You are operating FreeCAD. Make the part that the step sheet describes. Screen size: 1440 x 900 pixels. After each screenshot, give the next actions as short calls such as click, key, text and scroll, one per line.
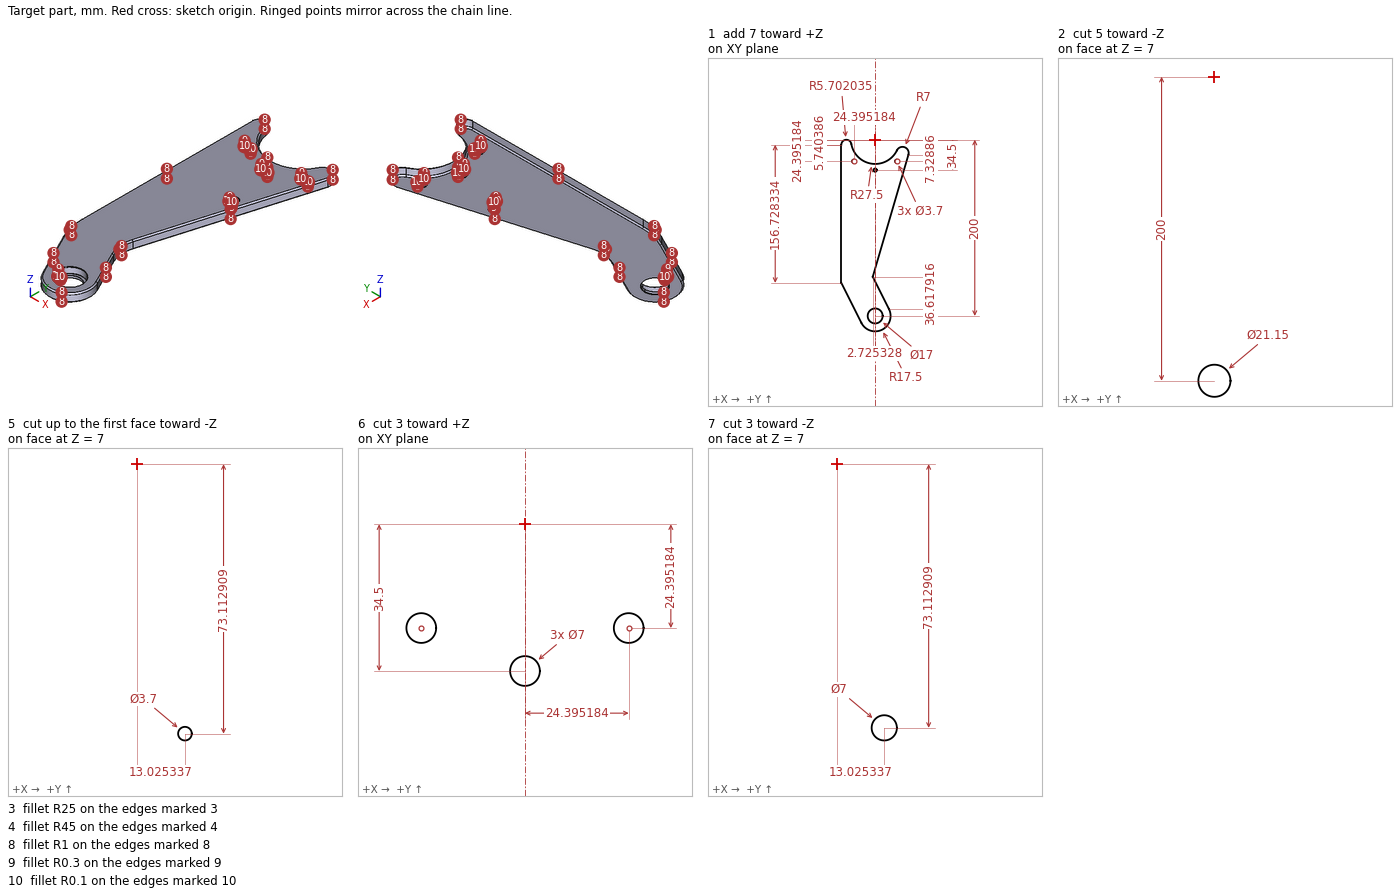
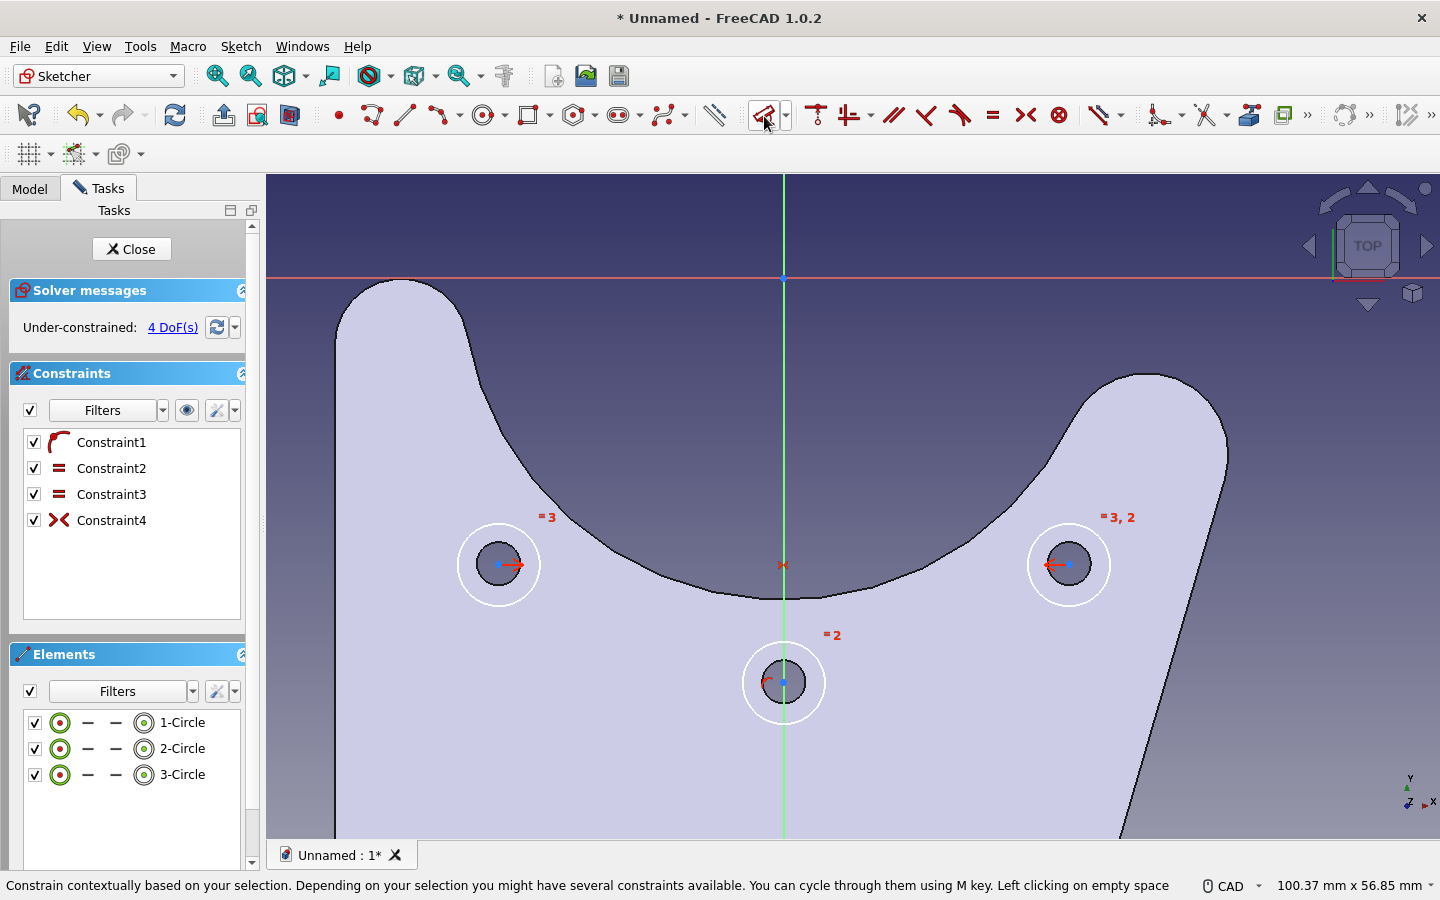
click(813, 654)
click(836, 631)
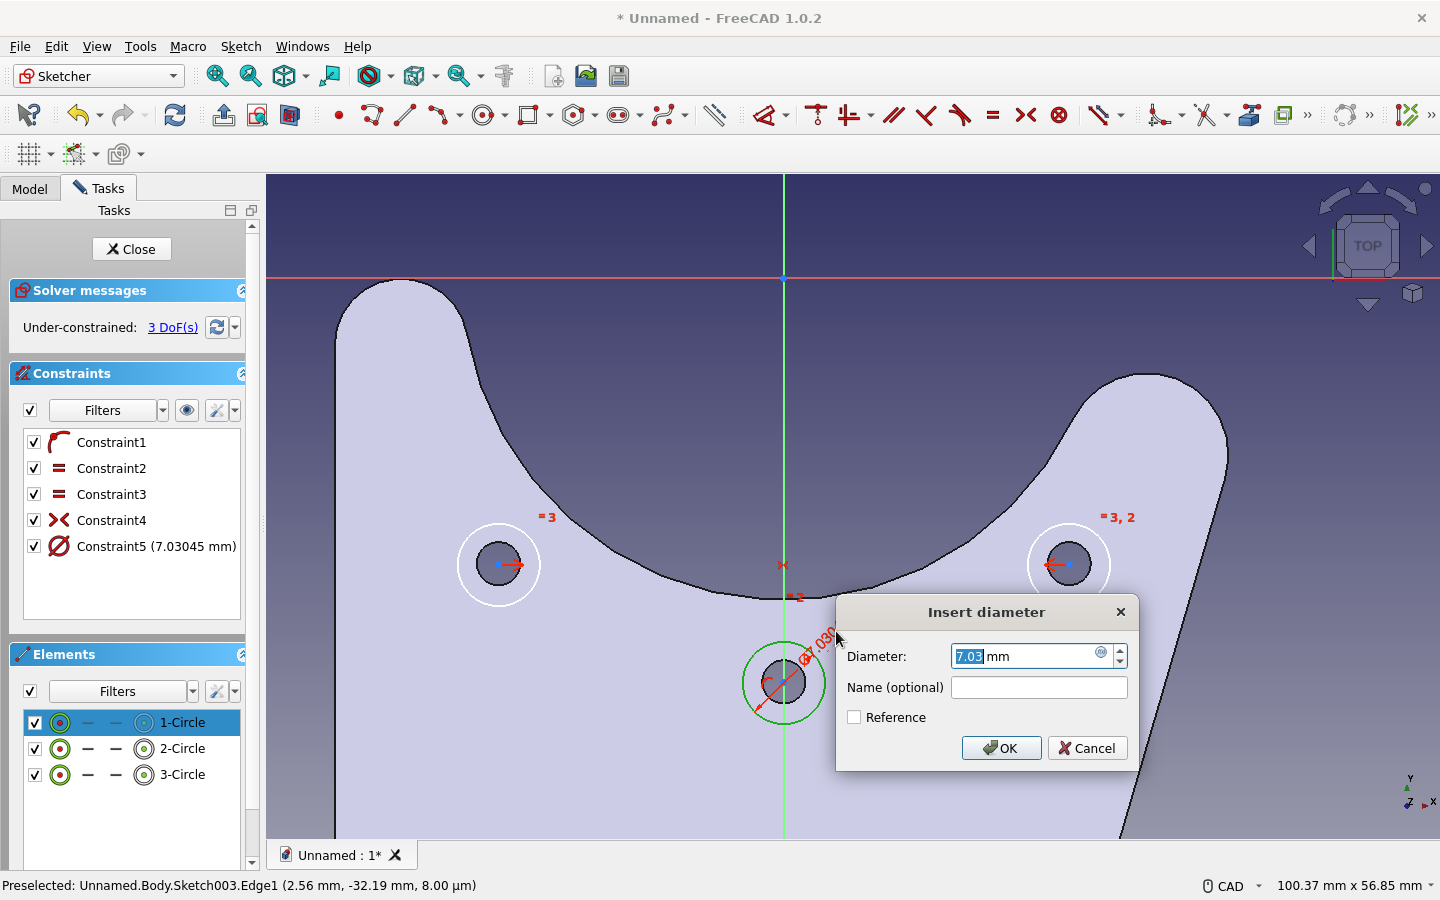
text(7)
key(Return)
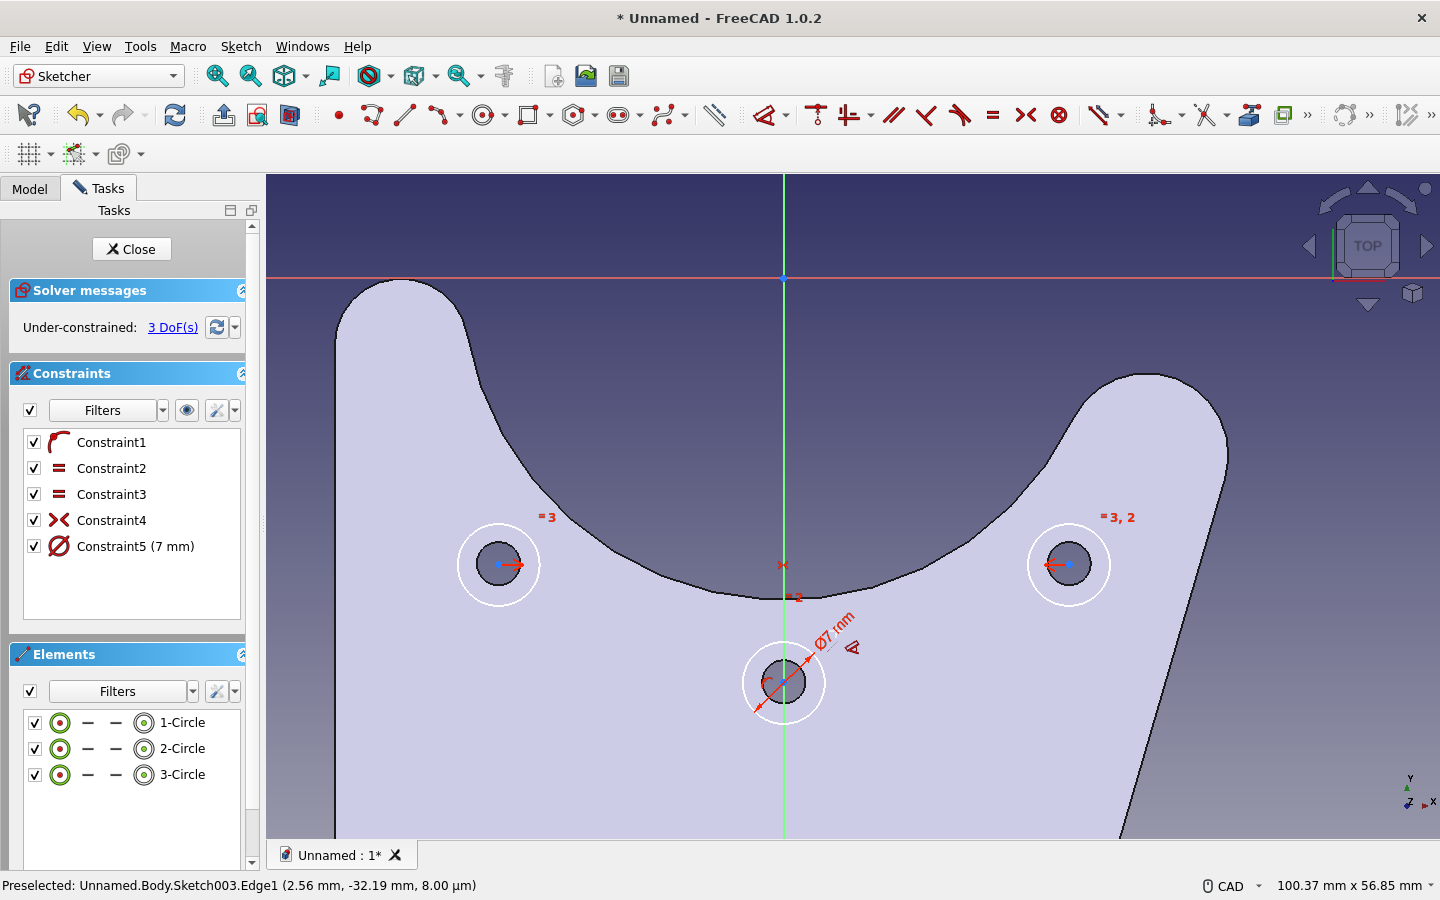
click(784, 683)
click(818, 481)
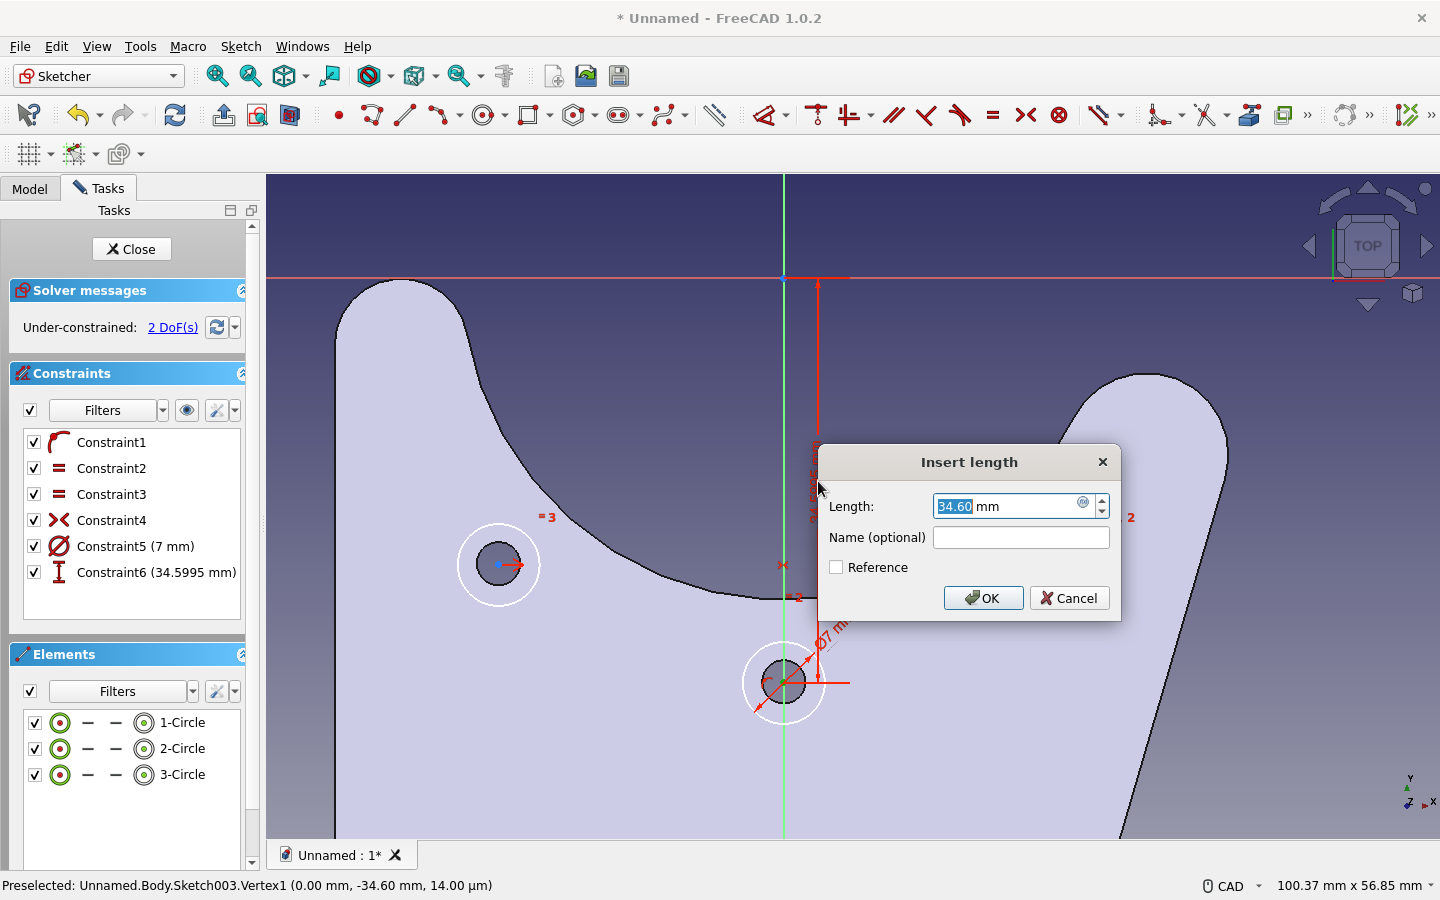
text(34.5)
key(Return)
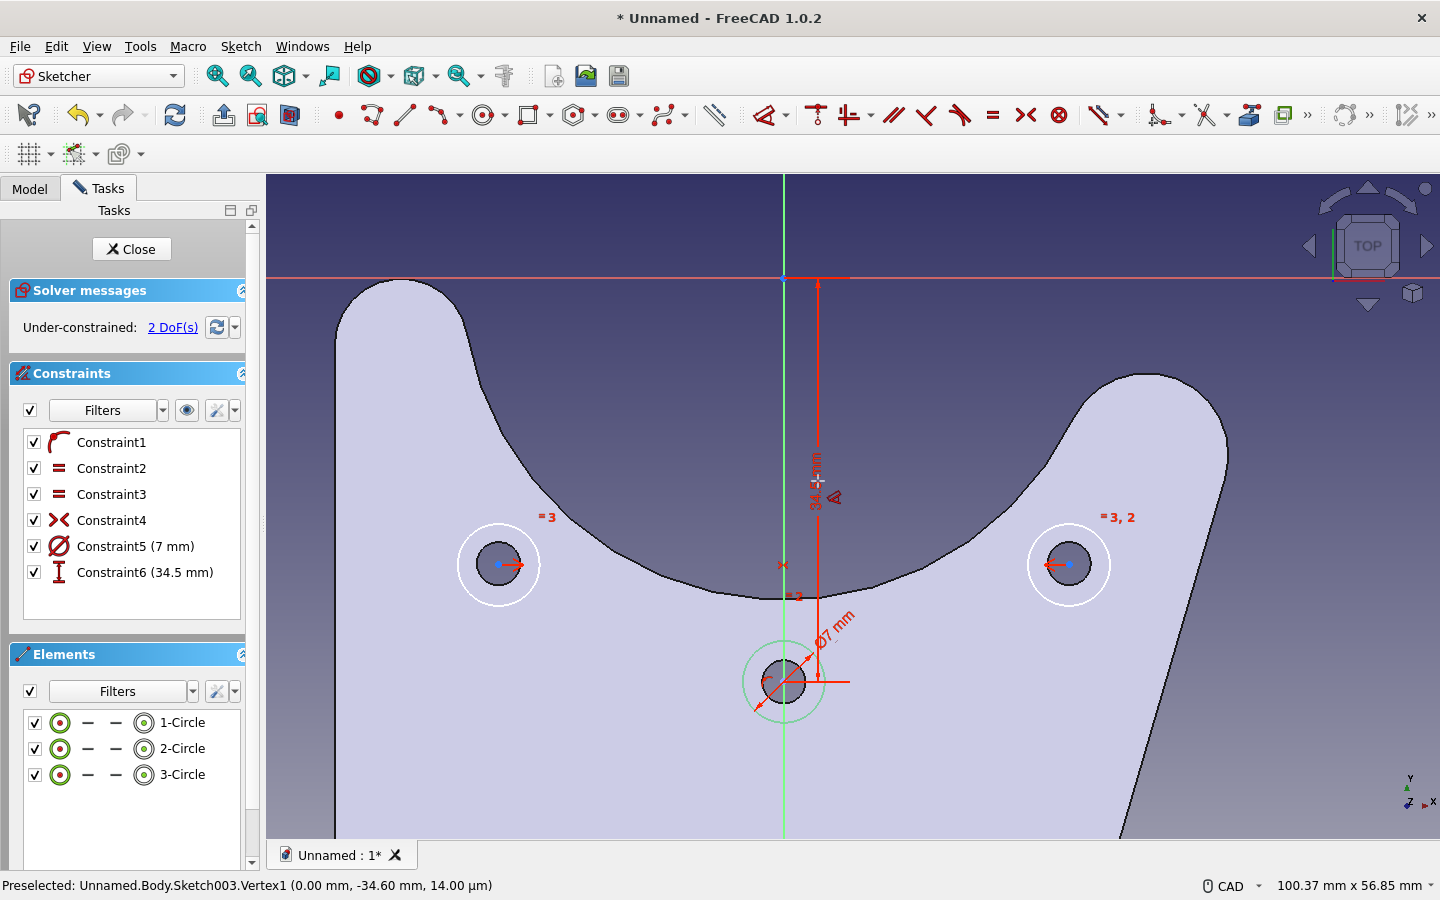
click(1069, 565)
click(926, 244)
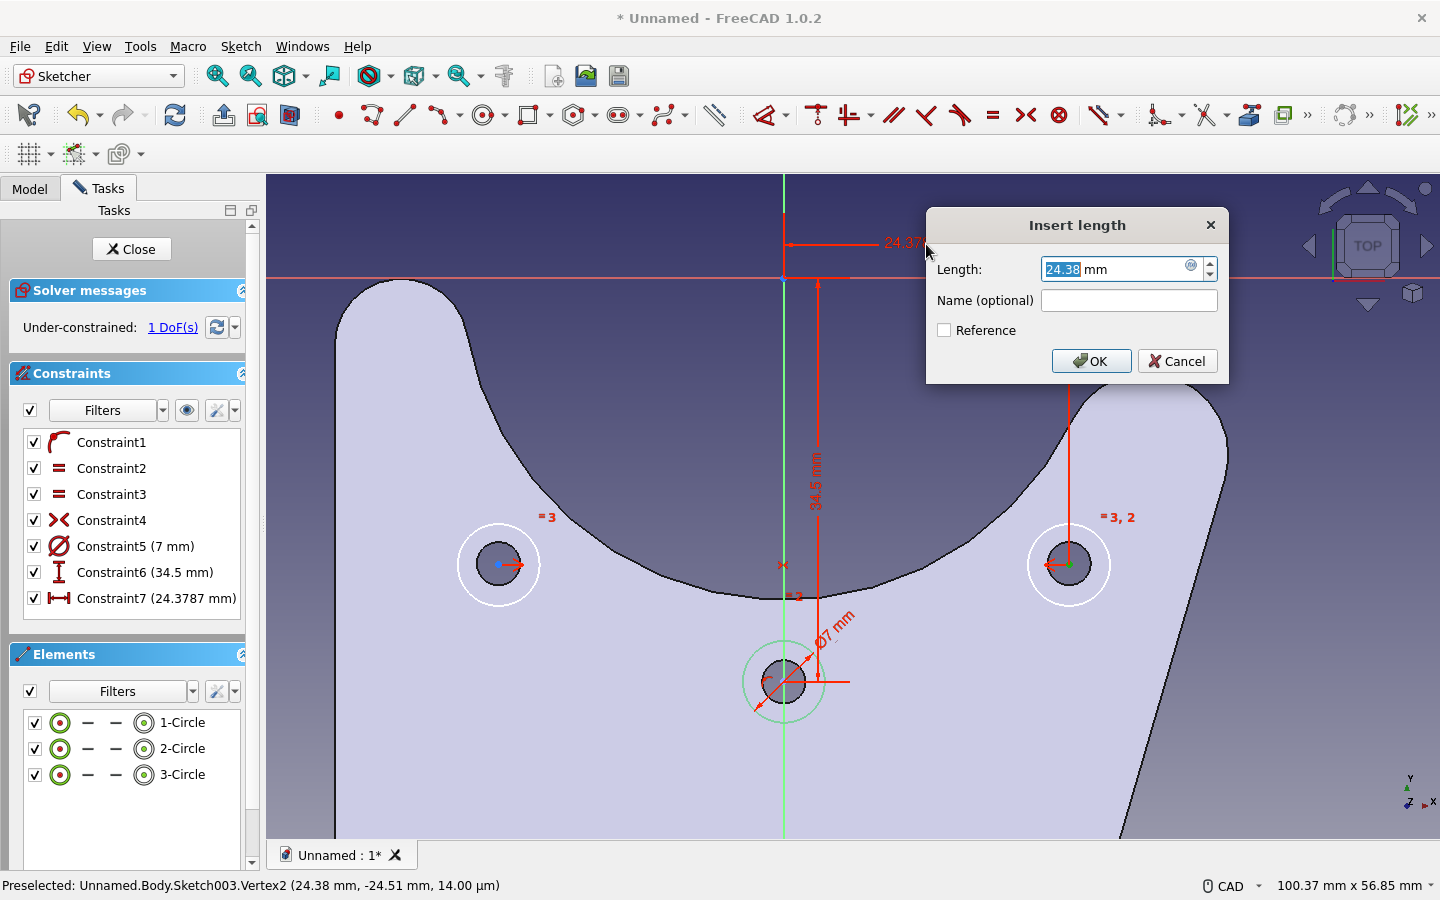
text(24.395184)
key(Return)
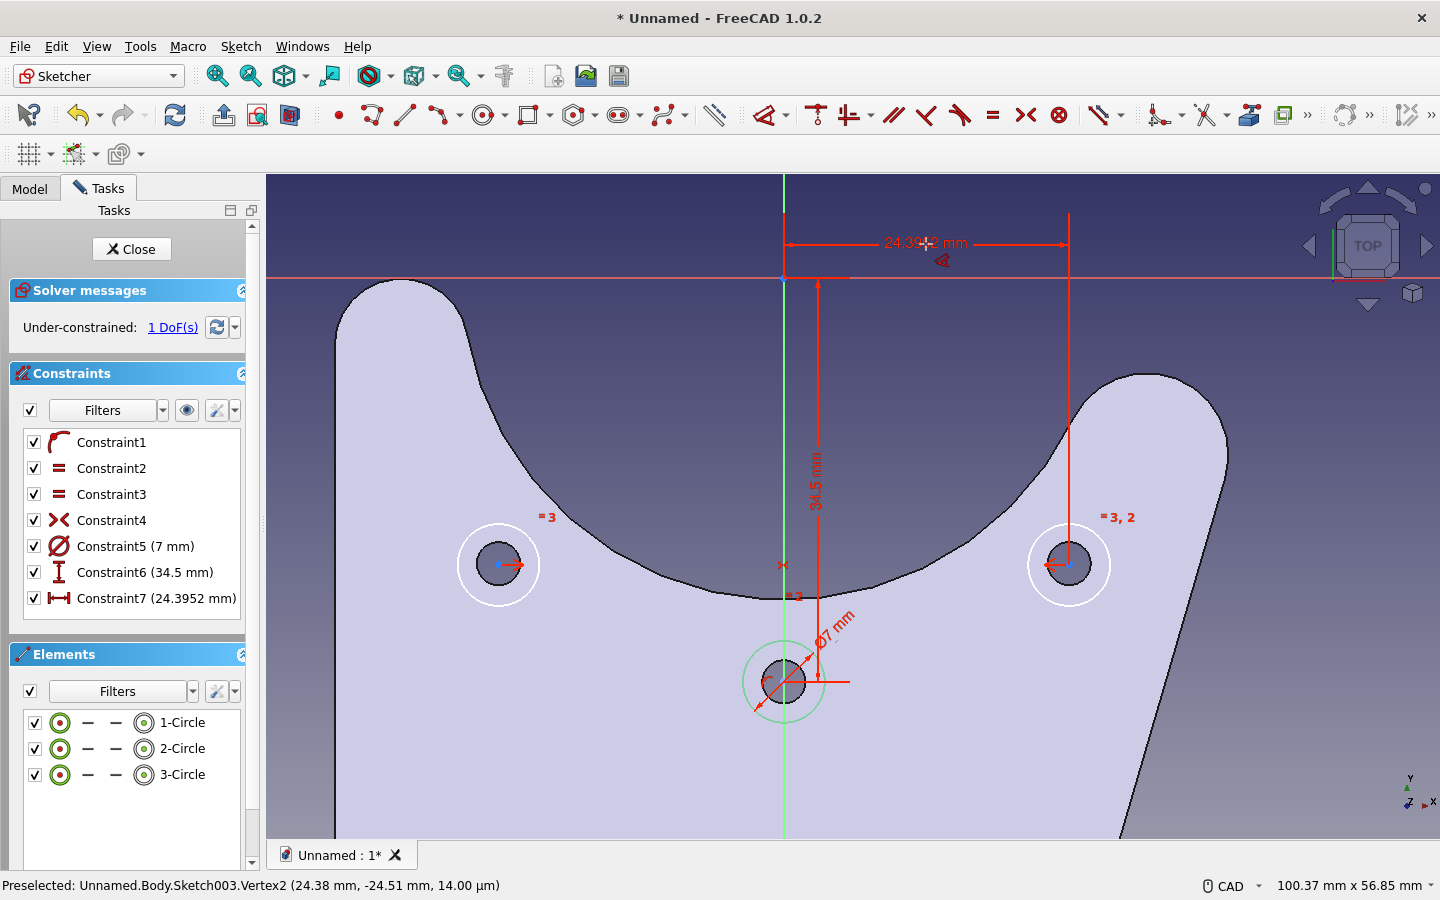
click(1069, 565)
click(1103, 422)